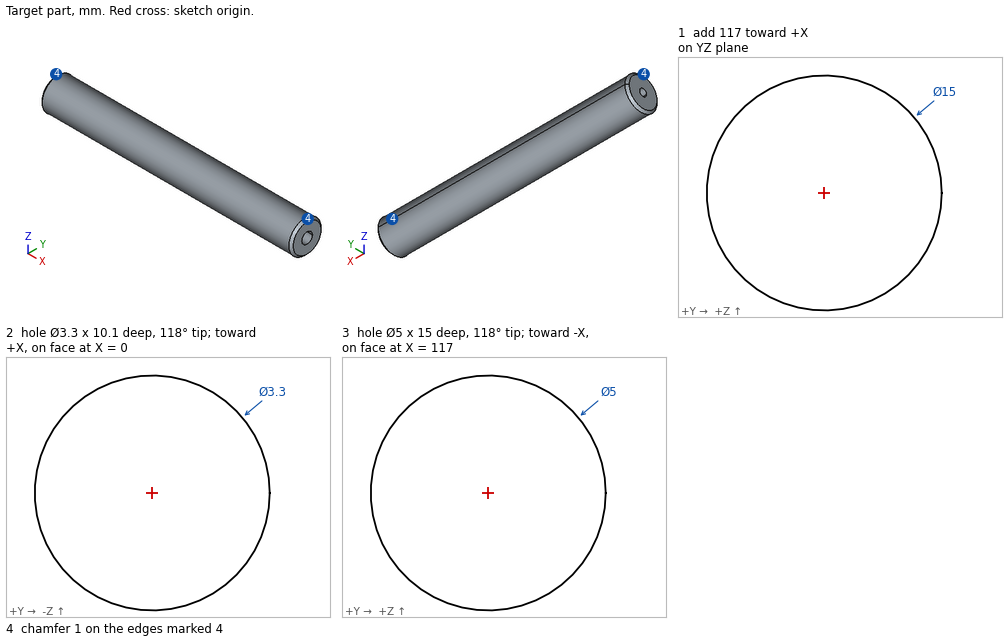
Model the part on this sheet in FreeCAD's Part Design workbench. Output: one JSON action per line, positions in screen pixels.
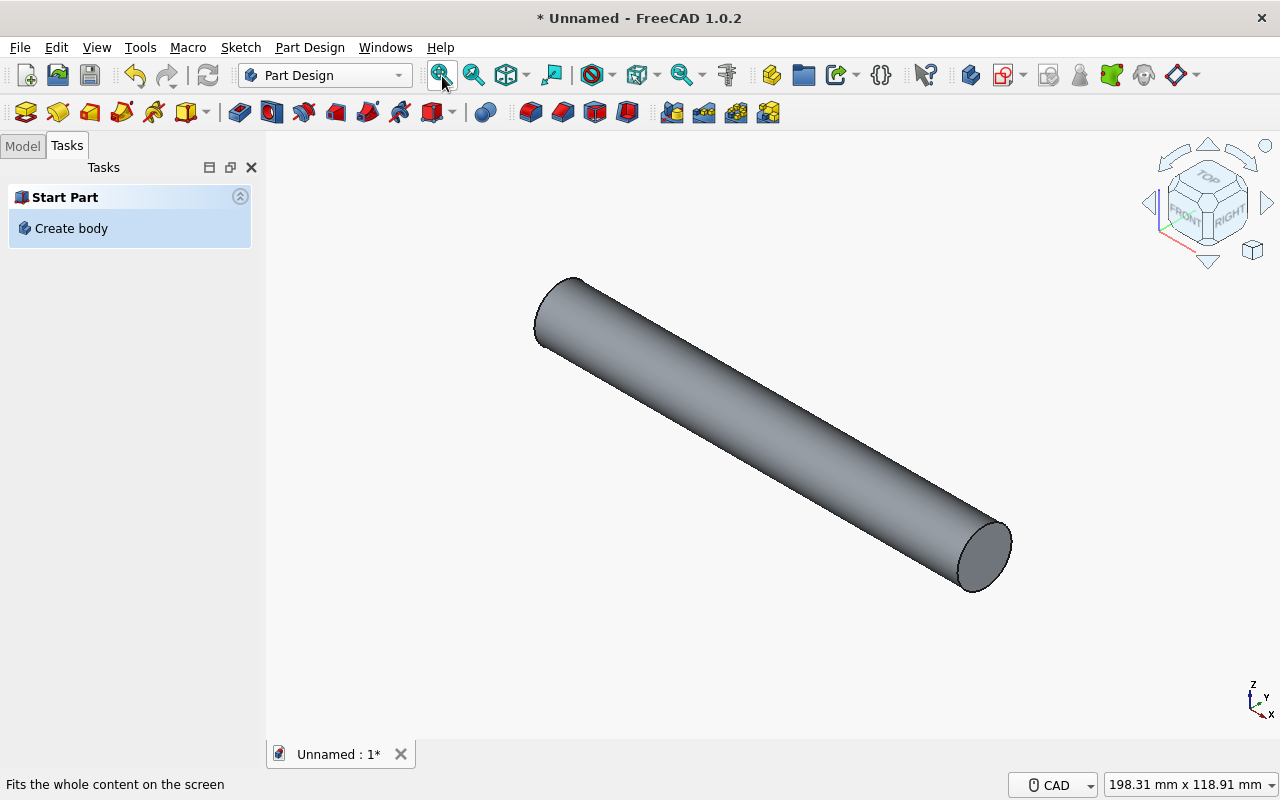
{"action": "left_click", "coordinate": [985, 556]}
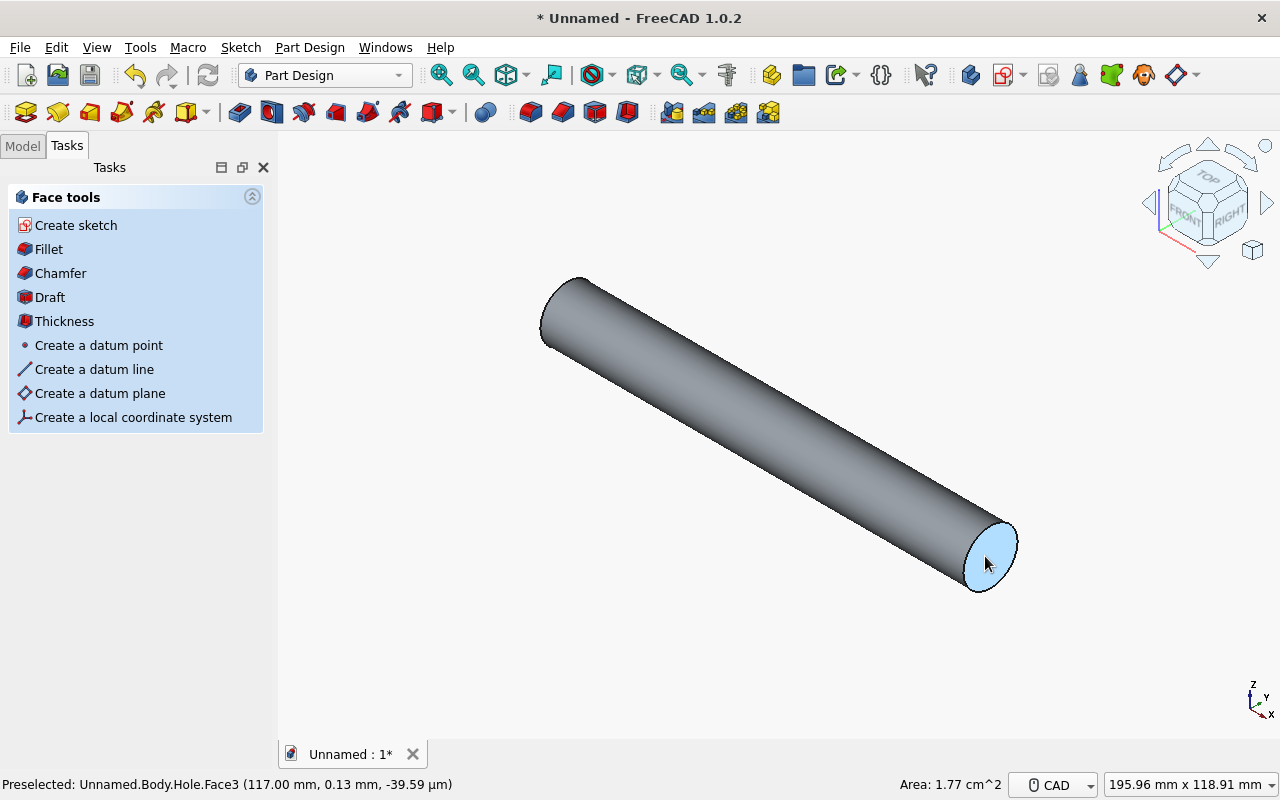
{"action": "left_click", "coordinate": [1004, 76]}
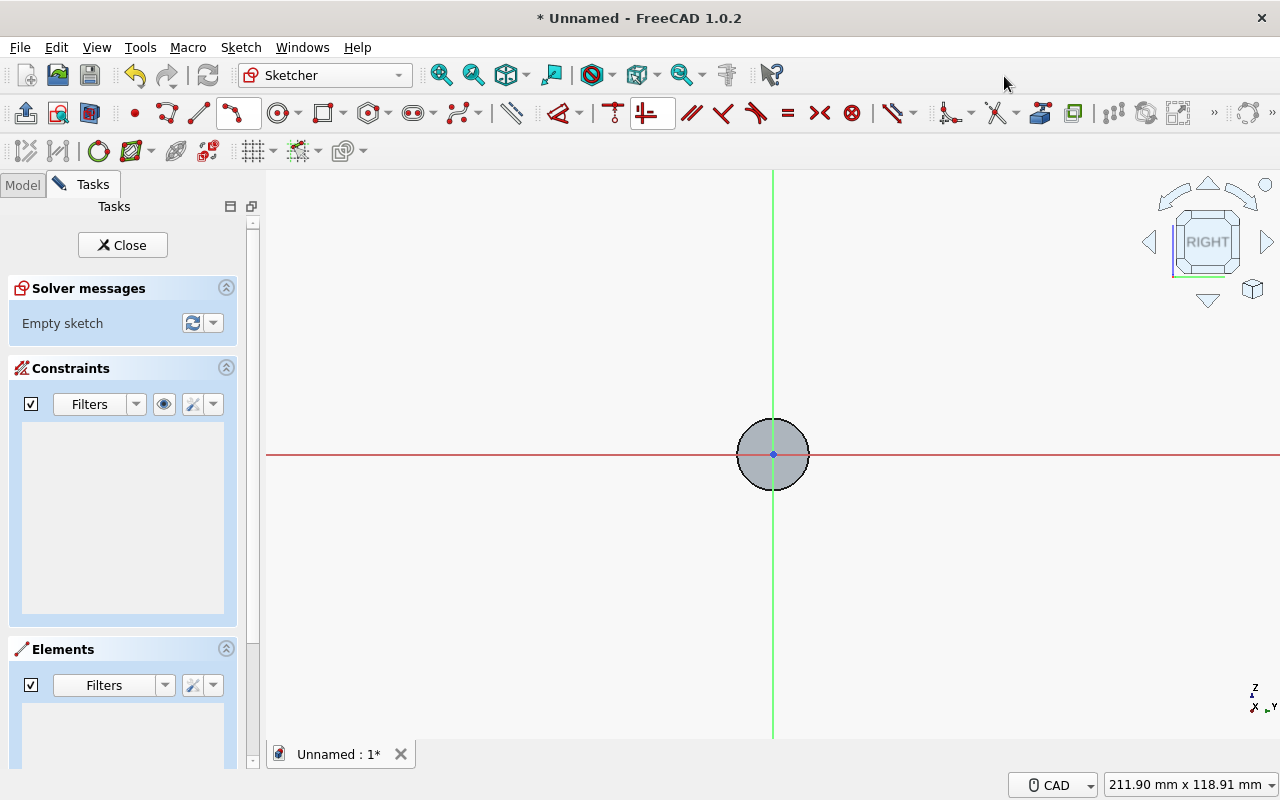
{"action": "scroll", "coordinate": [777, 454], "scroll_direction": "up", "scroll_amount": 14}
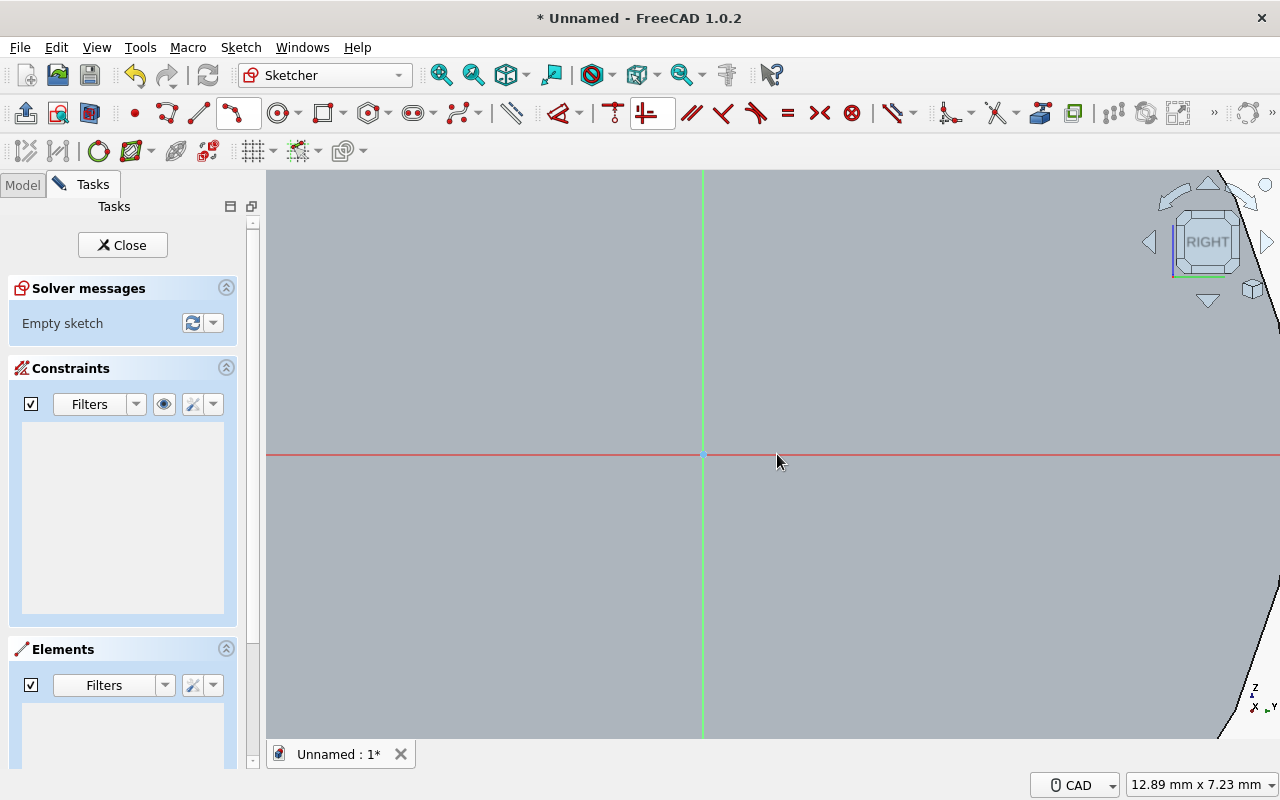
{"action": "left_click", "coordinate": [278, 114]}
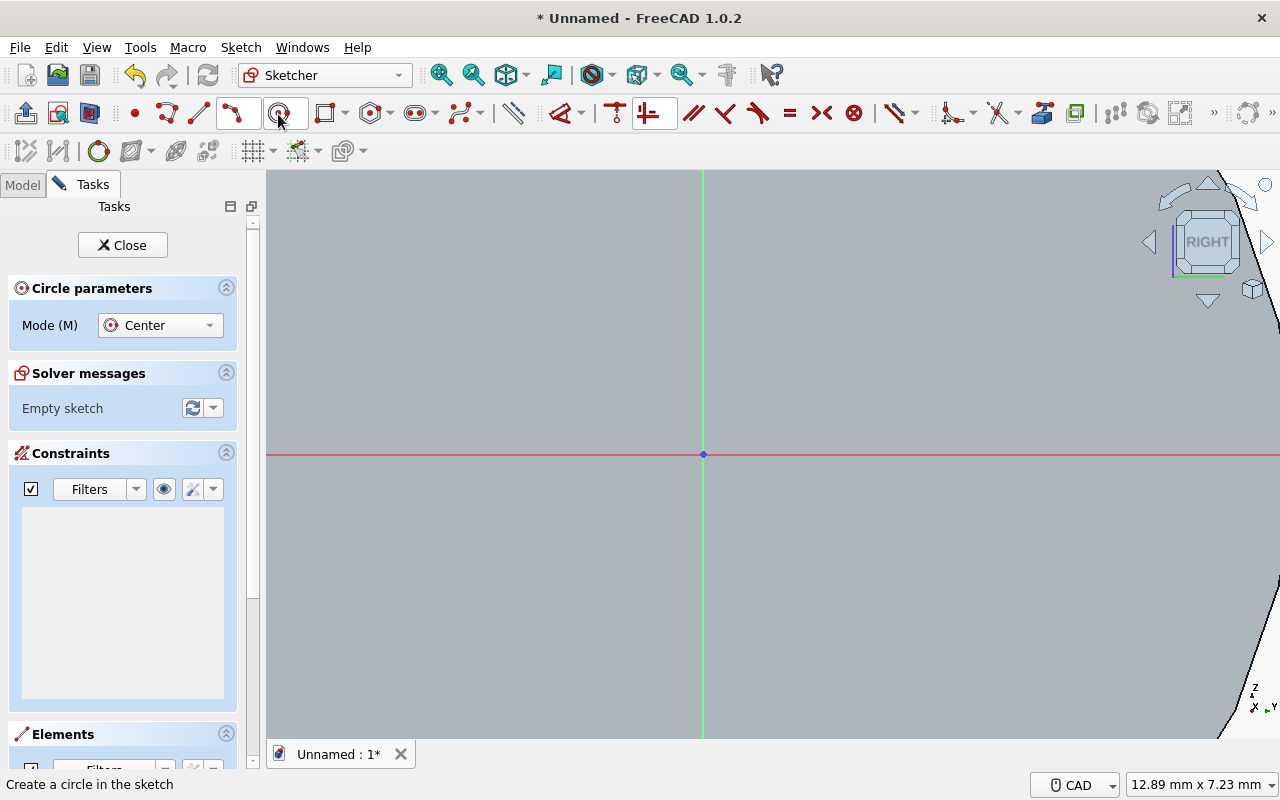
{"action": "left_click", "coordinate": [703, 454]}
{"action": "mouse_move", "coordinate": [843, 315]}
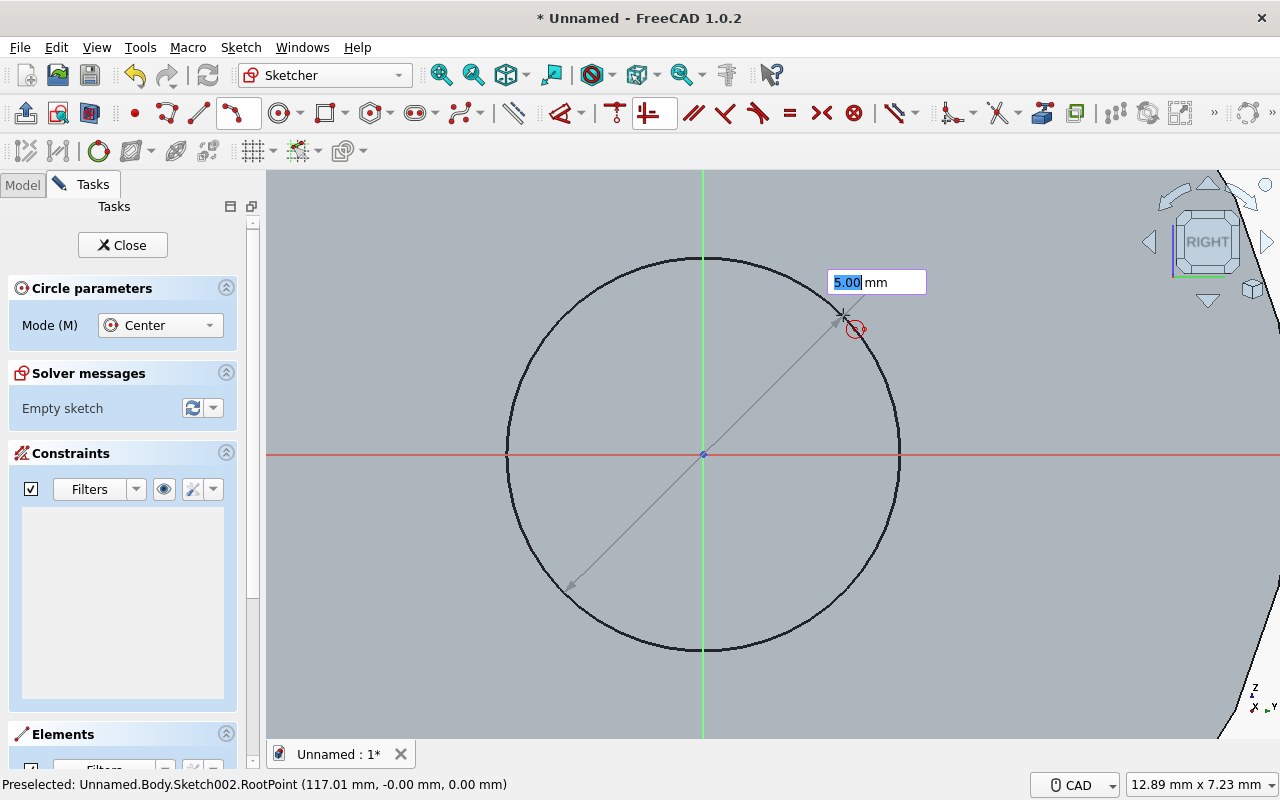
{"action": "type", "text": "5"}
{"action": "key", "text": "Return"}
{"action": "key", "text": "Escape"}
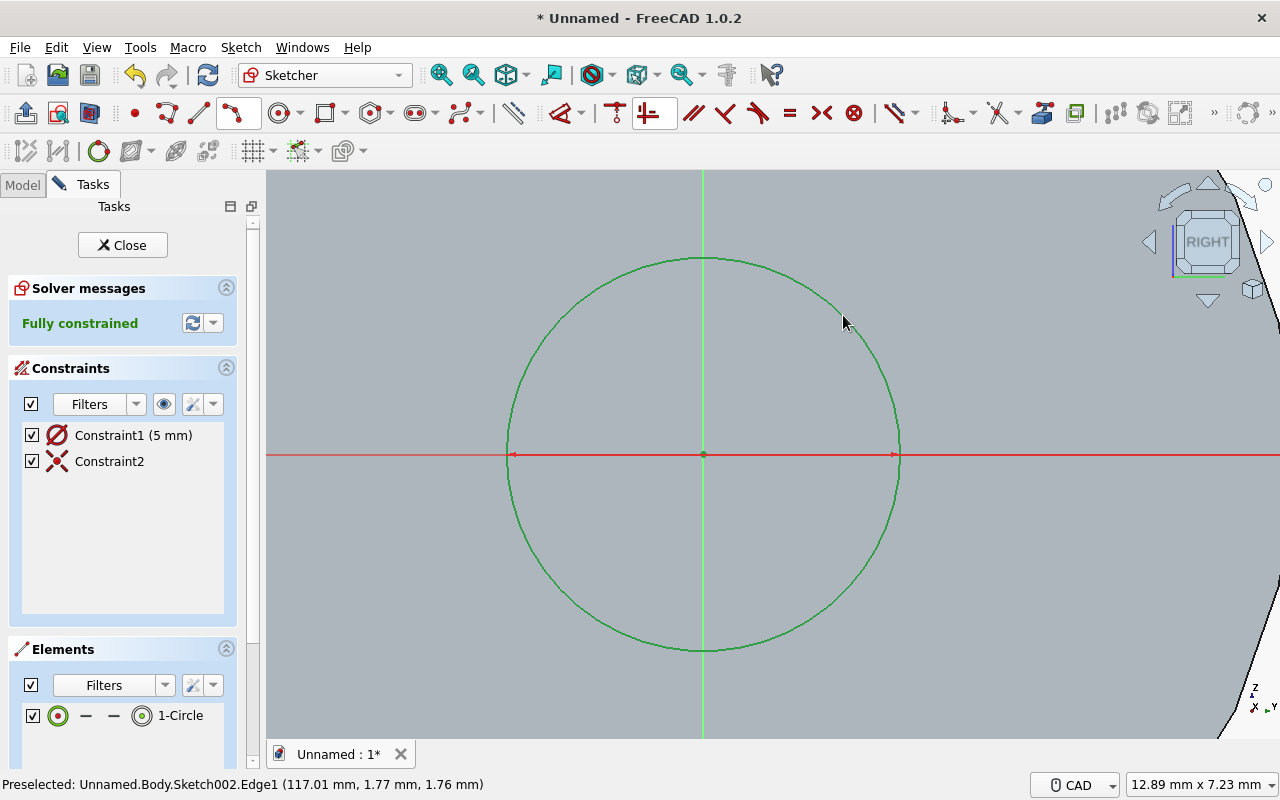
{"action": "left_click", "coordinate": [123, 245]}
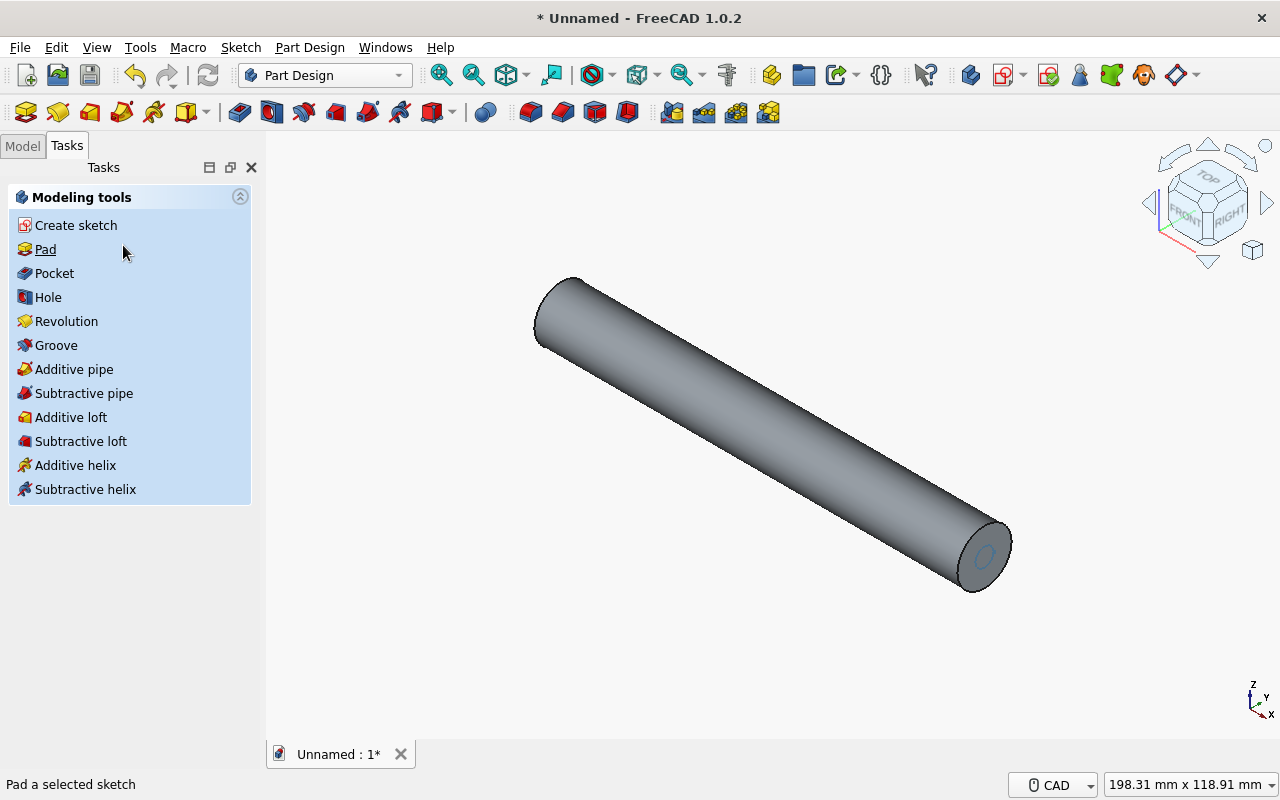
{"action": "left_click", "coordinate": [272, 112]}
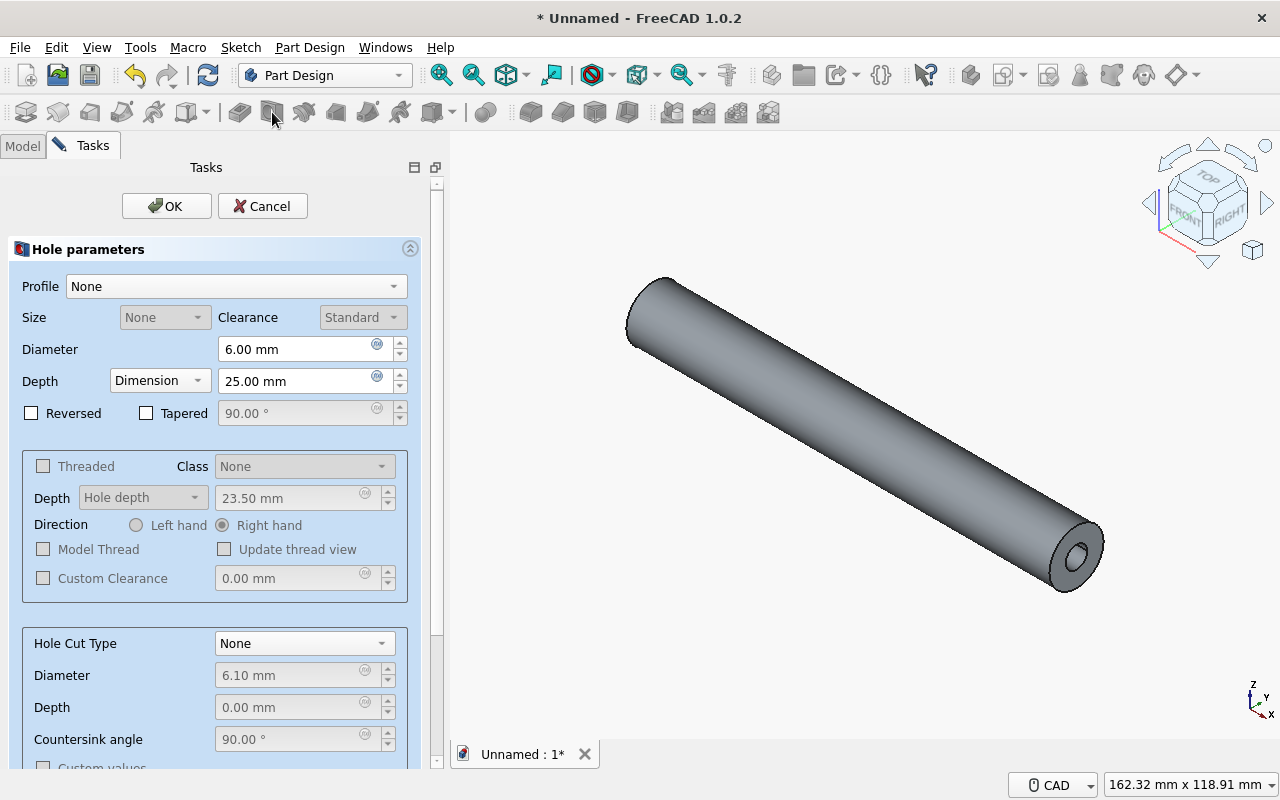
{"action": "triple_click", "coordinate": [305, 349]}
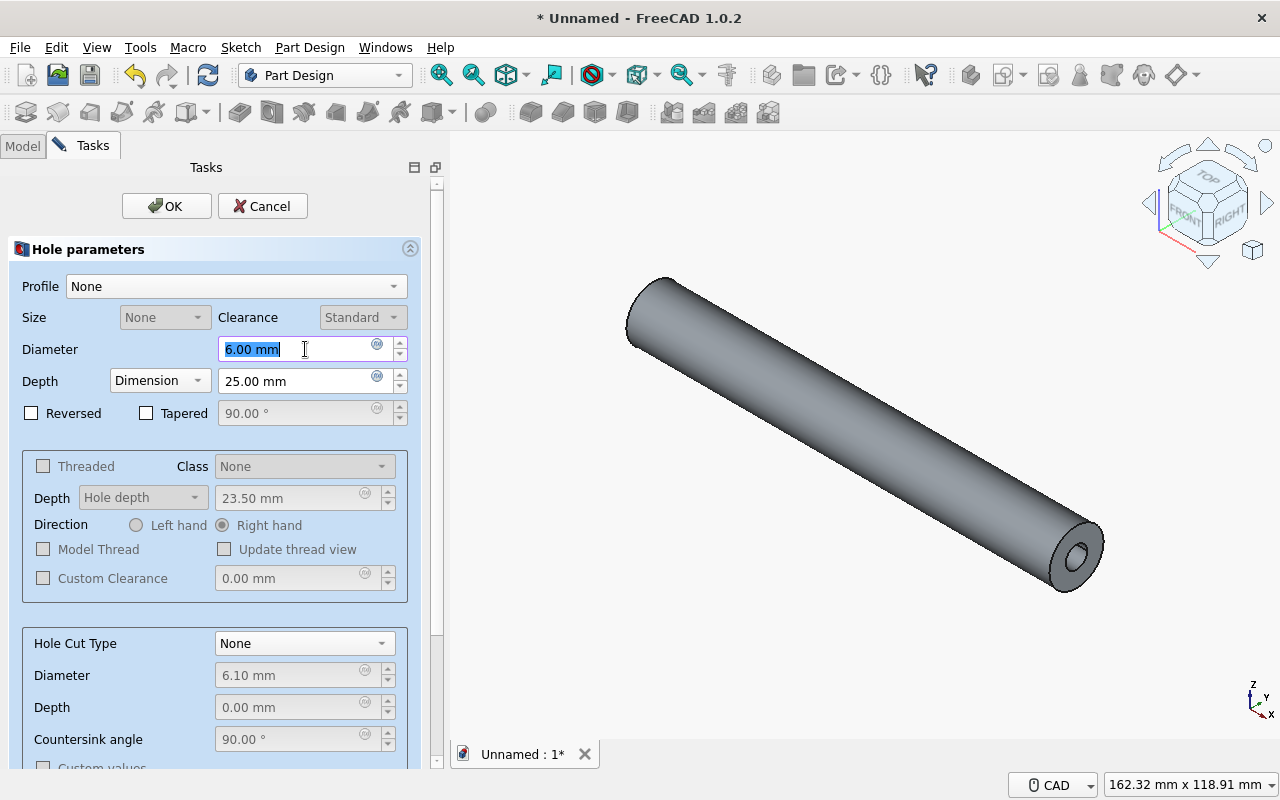
{"action": "type", "text": "5"}
{"action": "key", "text": "Tab"}